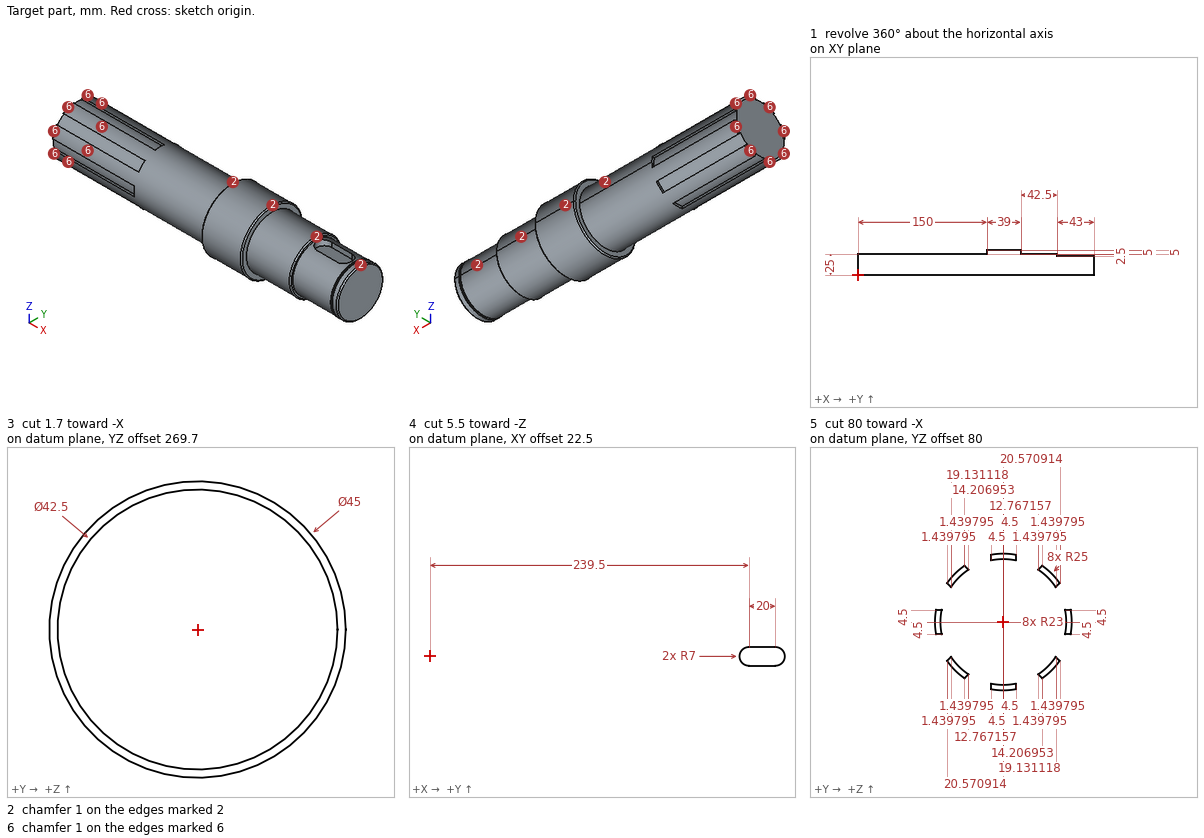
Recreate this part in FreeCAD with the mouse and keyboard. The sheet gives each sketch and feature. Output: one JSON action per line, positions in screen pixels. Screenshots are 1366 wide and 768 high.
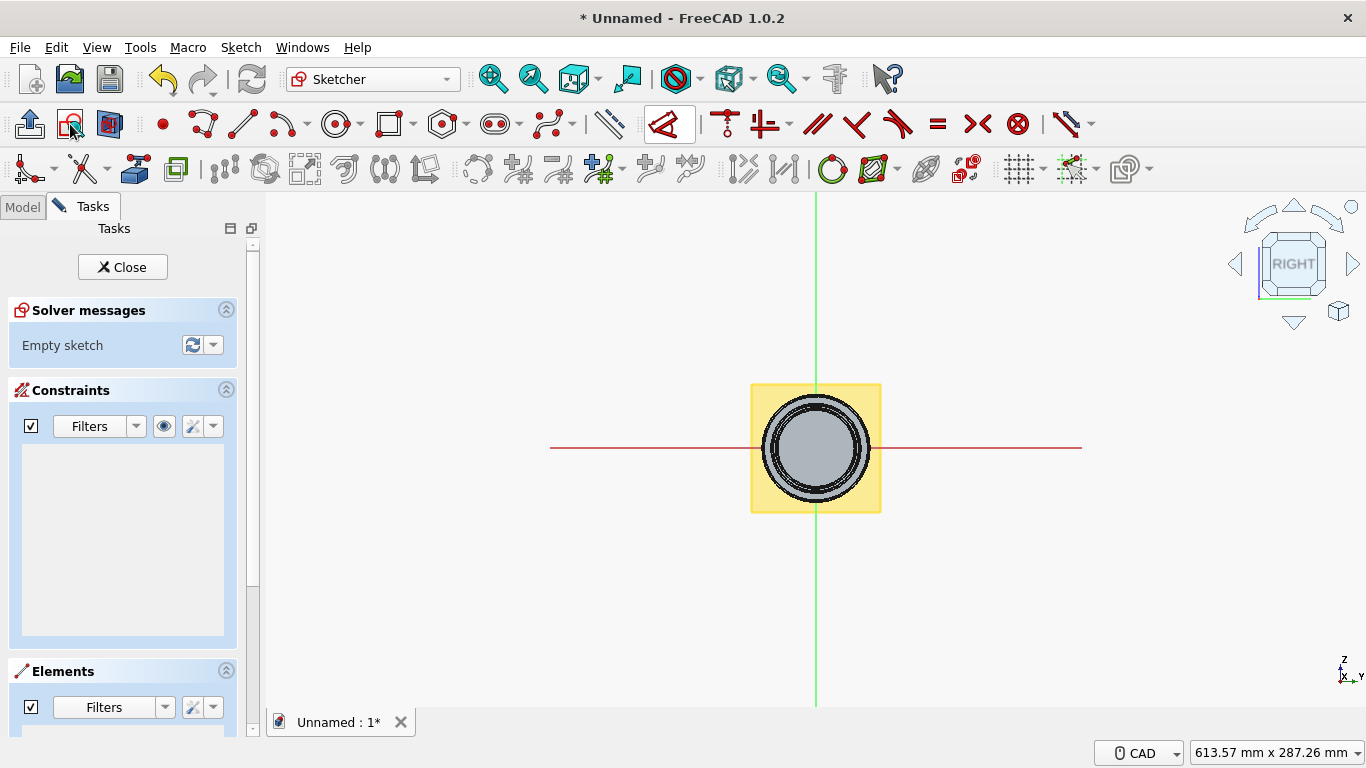
{"action": "left_click", "coordinate": [110, 124]}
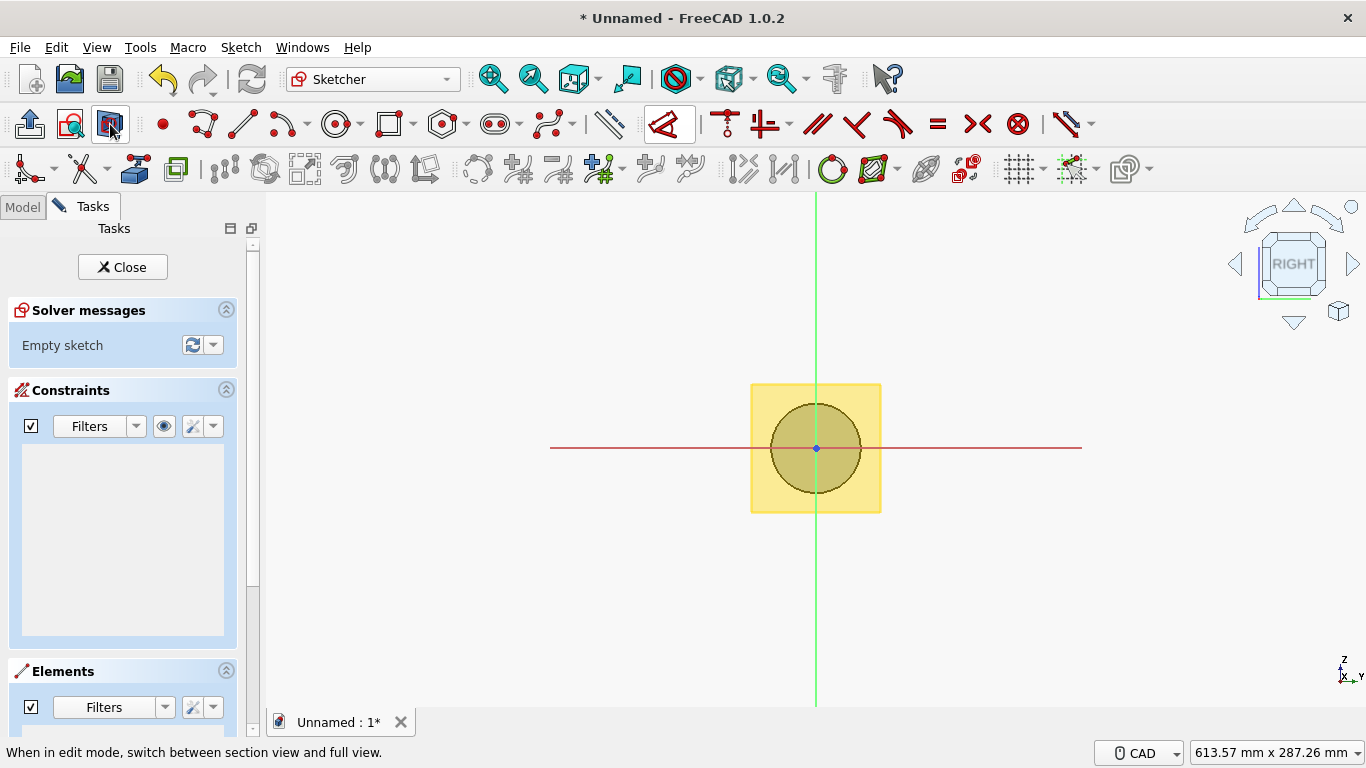
{"action": "scroll", "coordinate": [846, 448], "scroll_direction": "up", "scroll_amount": 6}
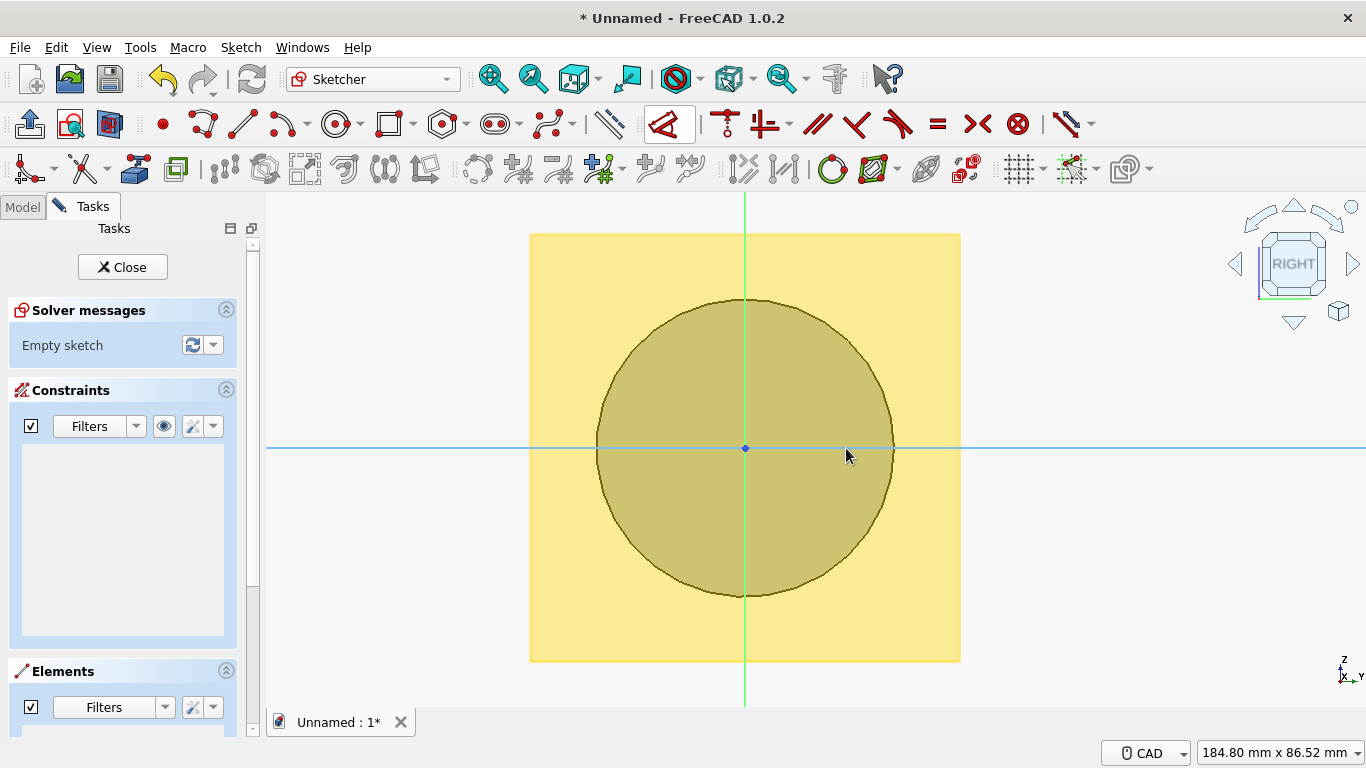
{"action": "left_click", "coordinate": [244, 124]}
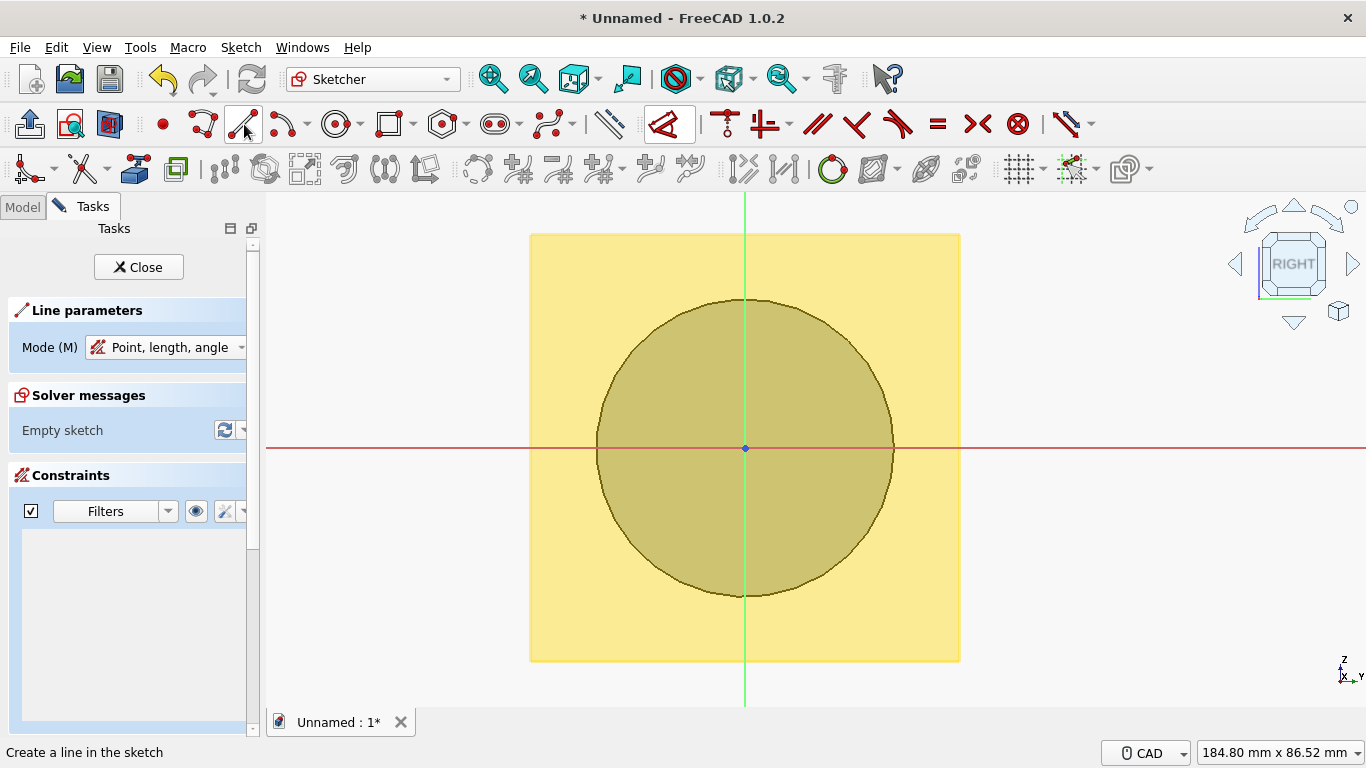
{"action": "left_click", "coordinate": [892, 475]}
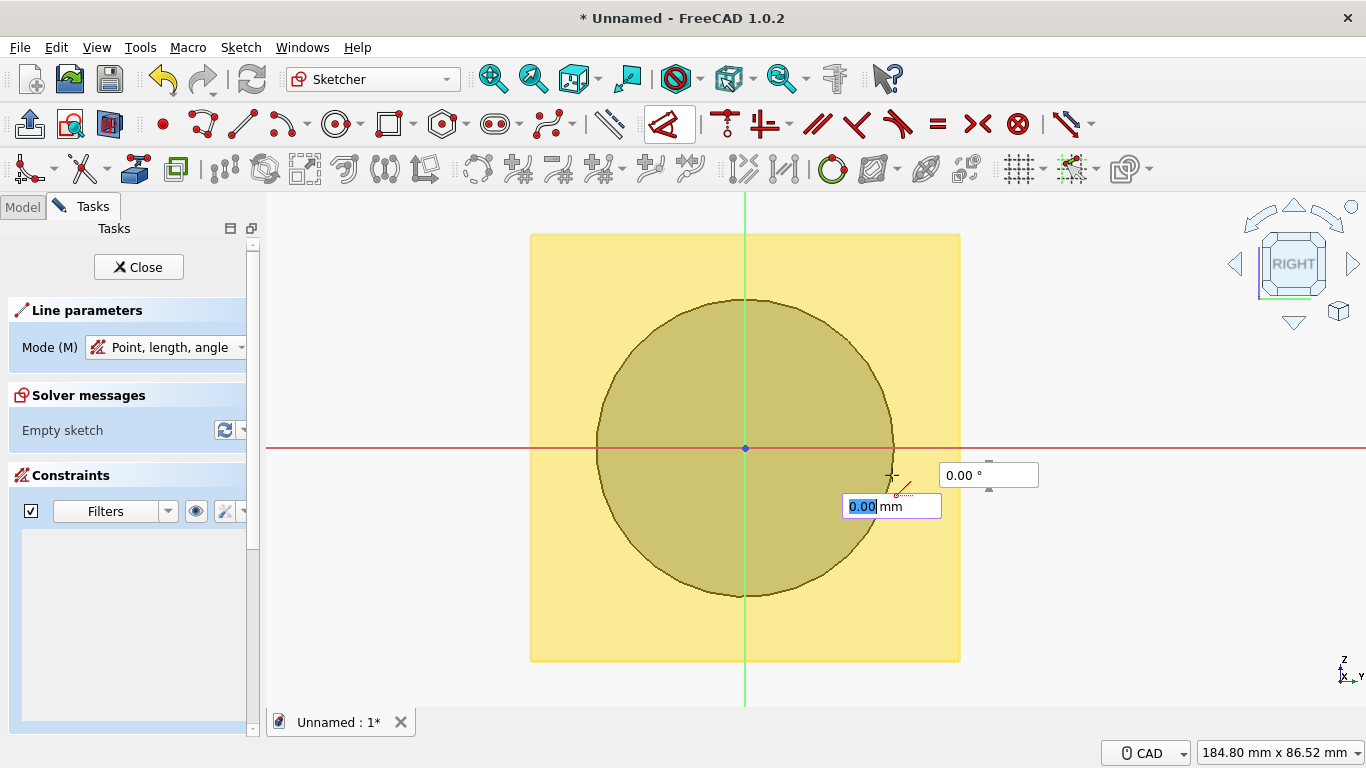
{"action": "scroll", "coordinate": [879, 475], "scroll_direction": "up", "scroll_amount": 2}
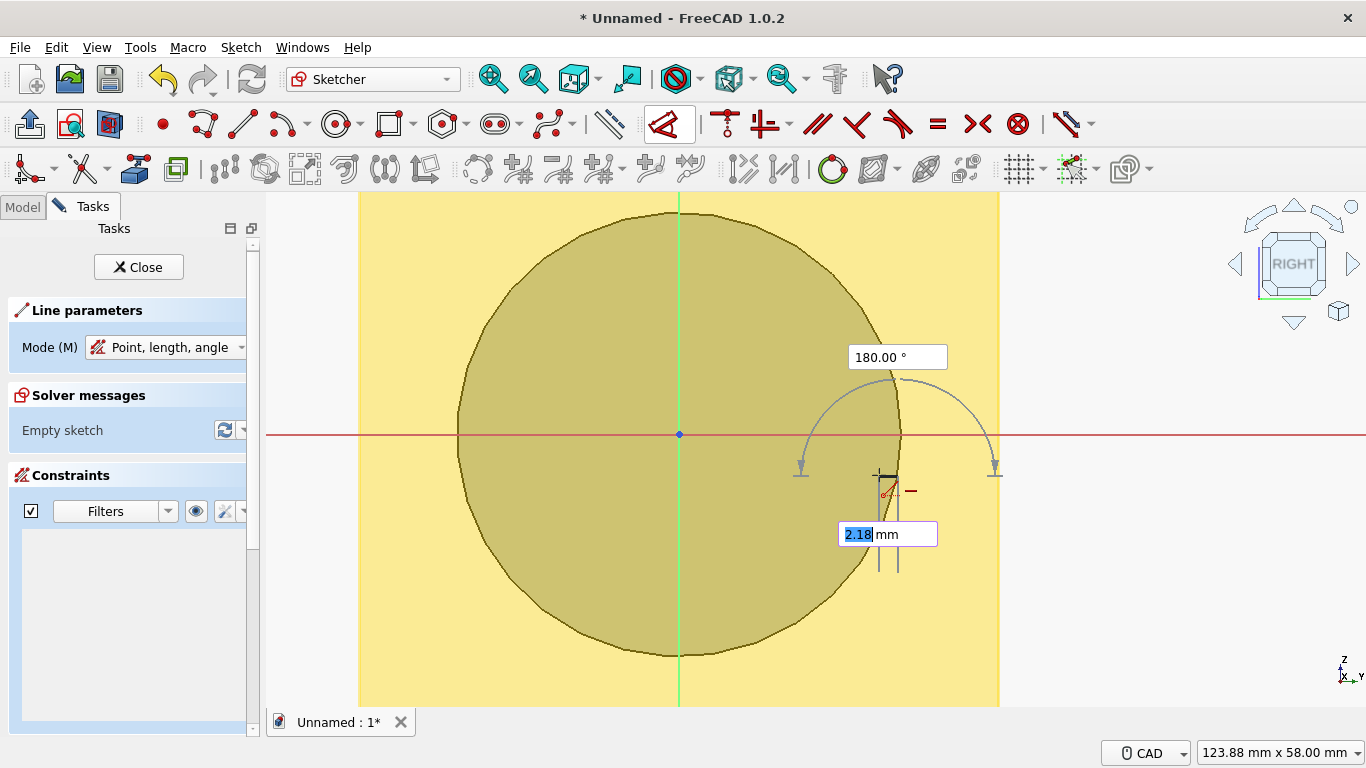
{"action": "left_click", "coordinate": [879, 475]}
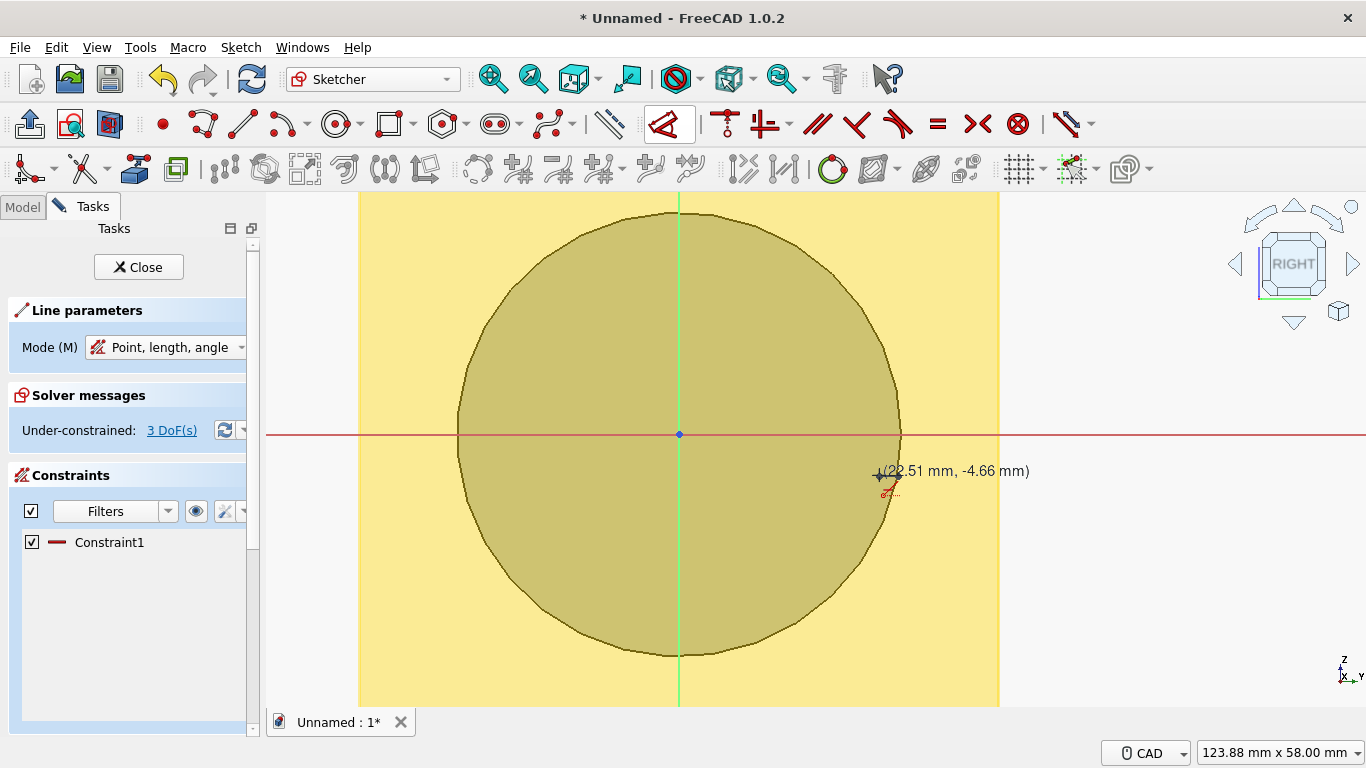
{"action": "left_click", "coordinate": [879, 395]}
{"action": "left_click", "coordinate": [897, 395]}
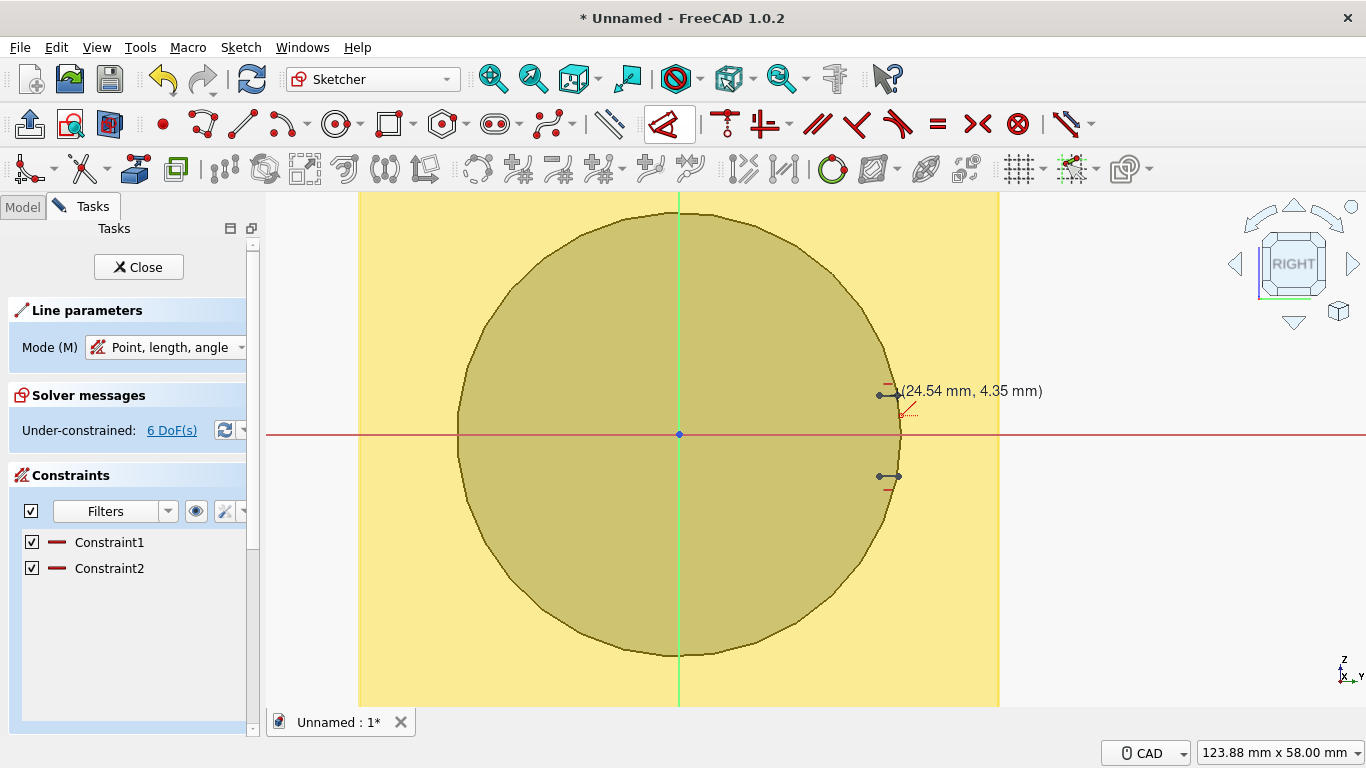
{"action": "key", "text": "g 3 a"}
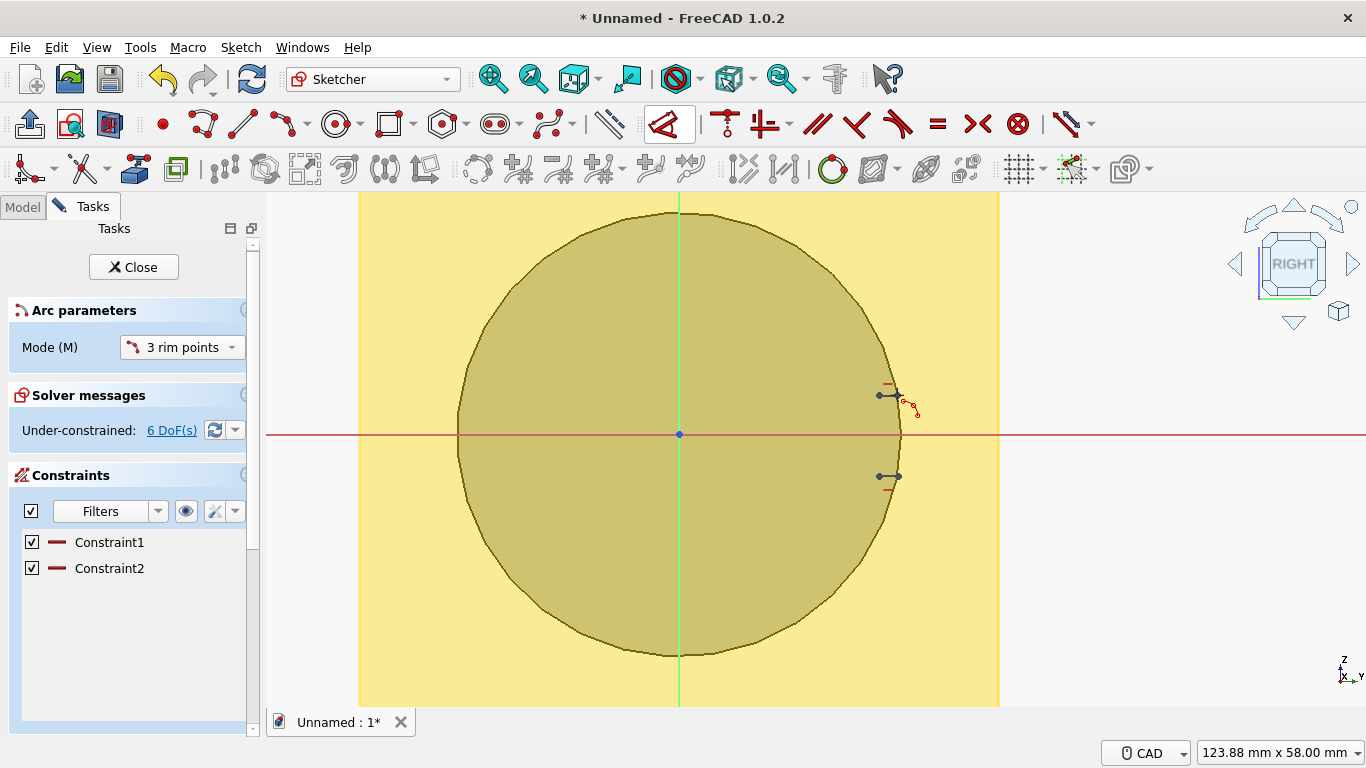
{"action": "scroll", "coordinate": [879, 475], "scroll_direction": "up", "scroll_amount": 3}